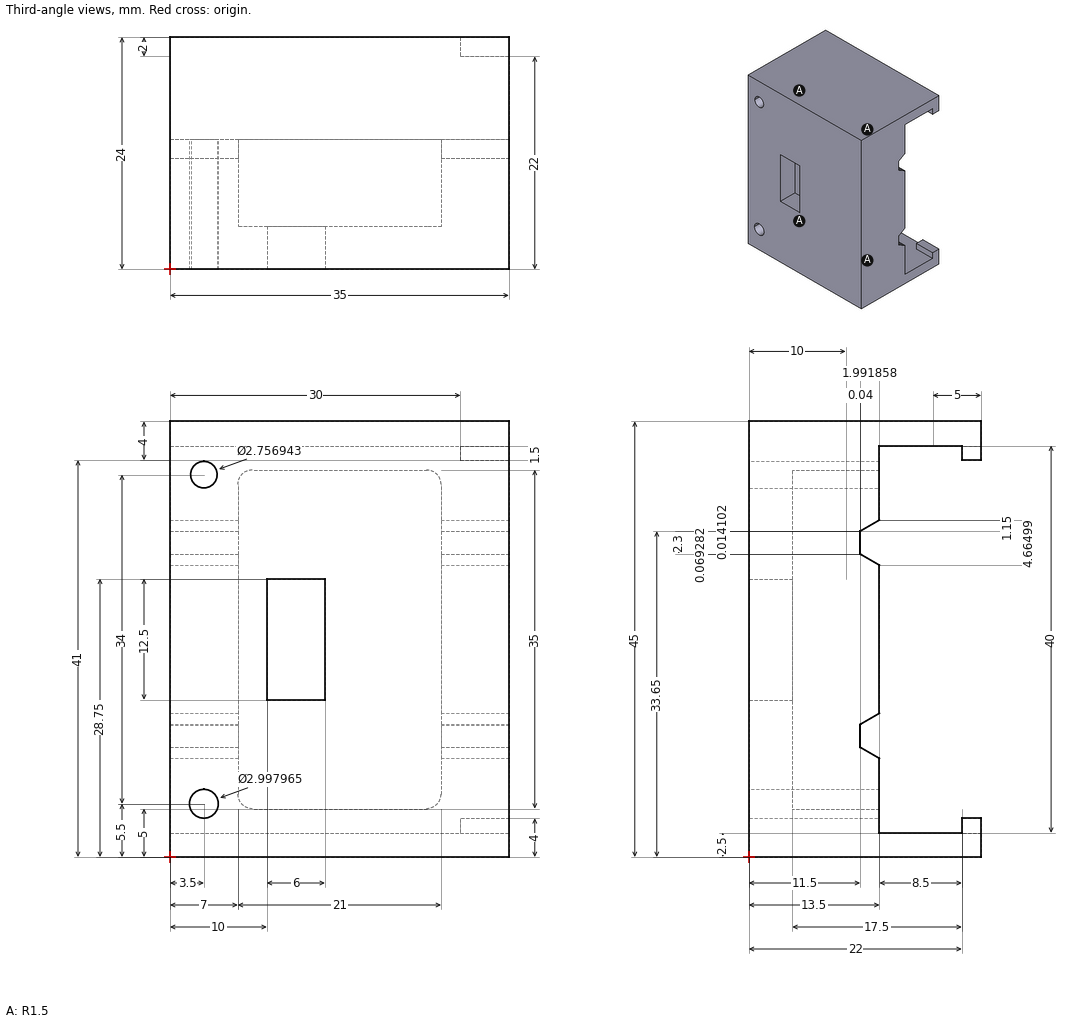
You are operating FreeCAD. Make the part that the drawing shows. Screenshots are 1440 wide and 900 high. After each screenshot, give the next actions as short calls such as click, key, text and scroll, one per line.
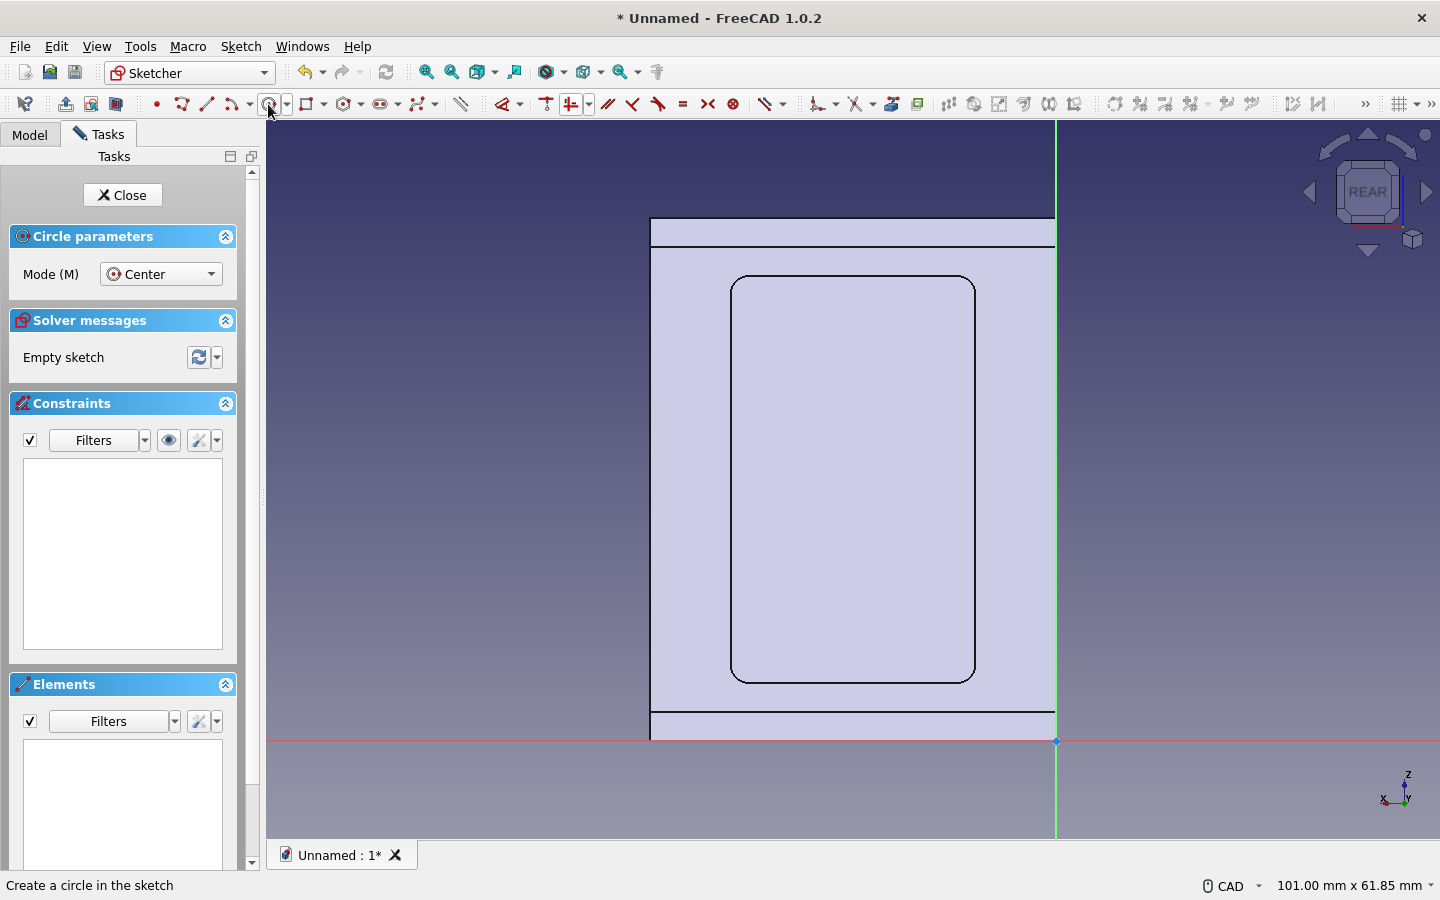
scroll(1016, 677, up, 2)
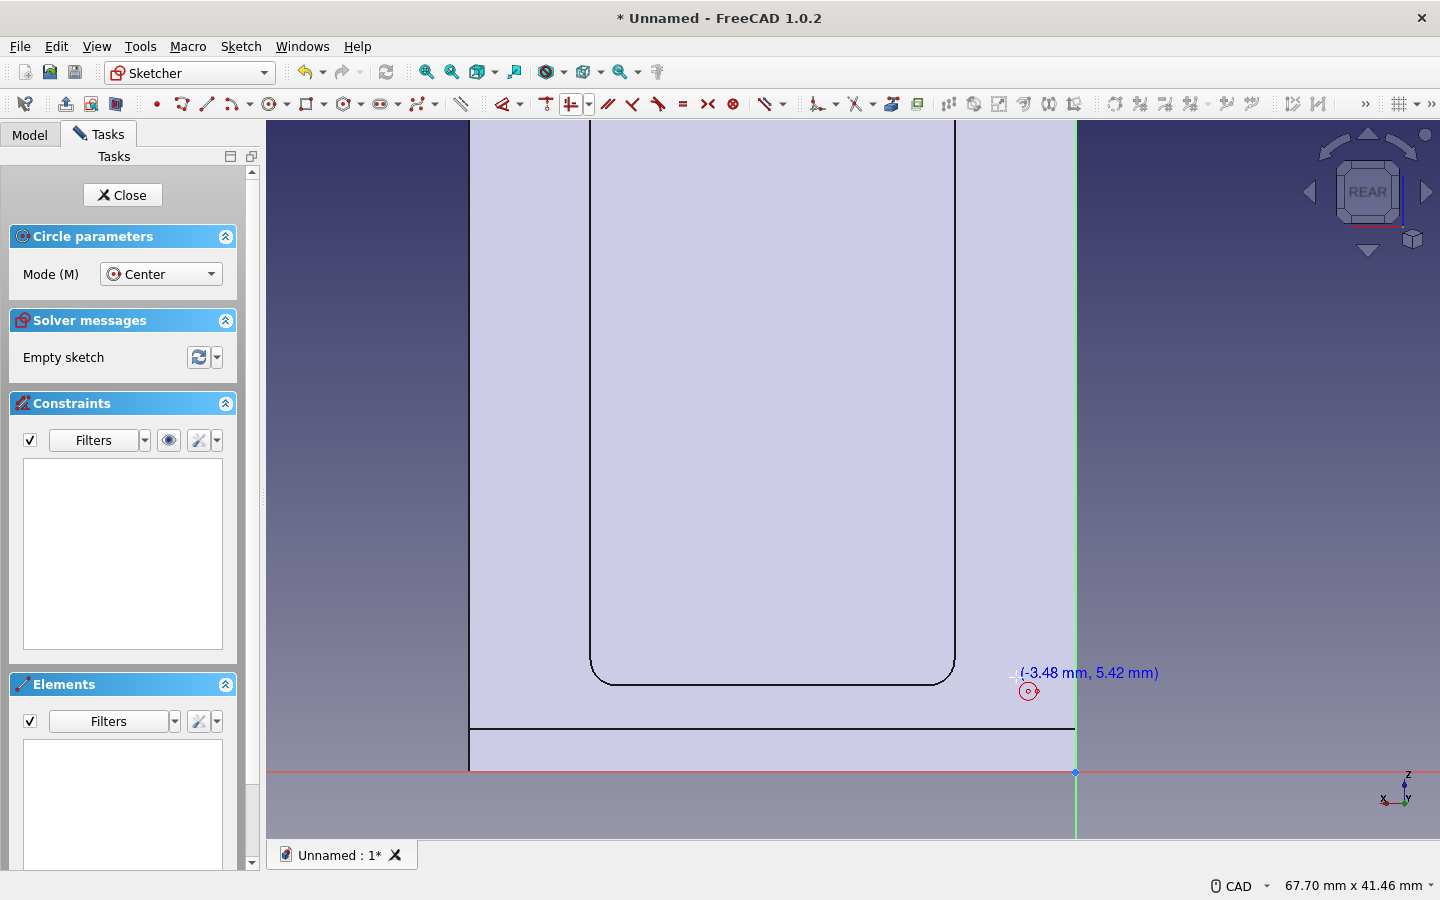
click(1015, 677)
click(1034, 658)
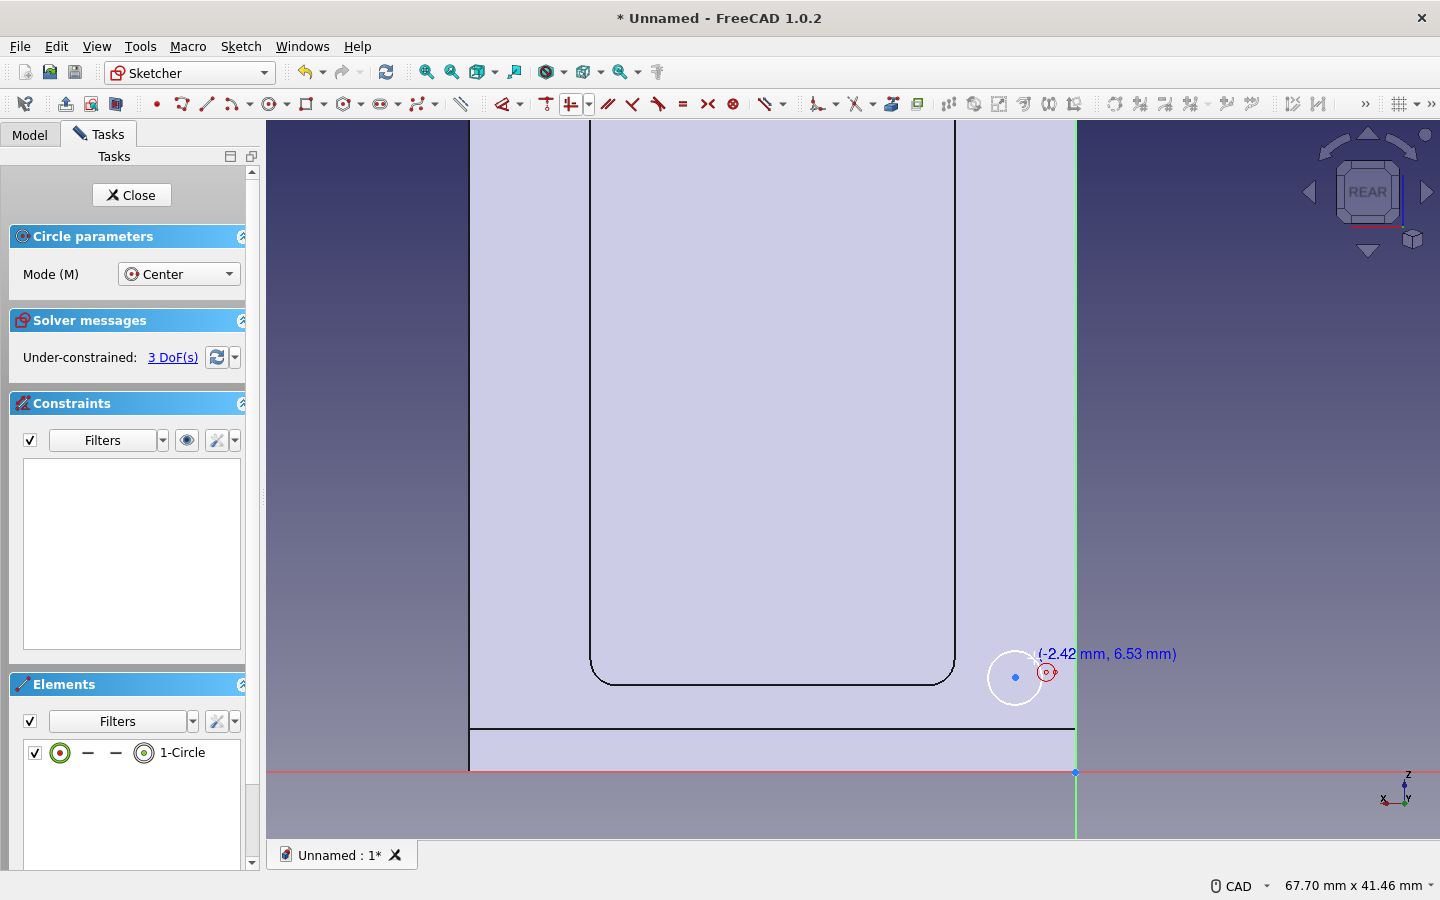
scroll(294, 605, down, 2)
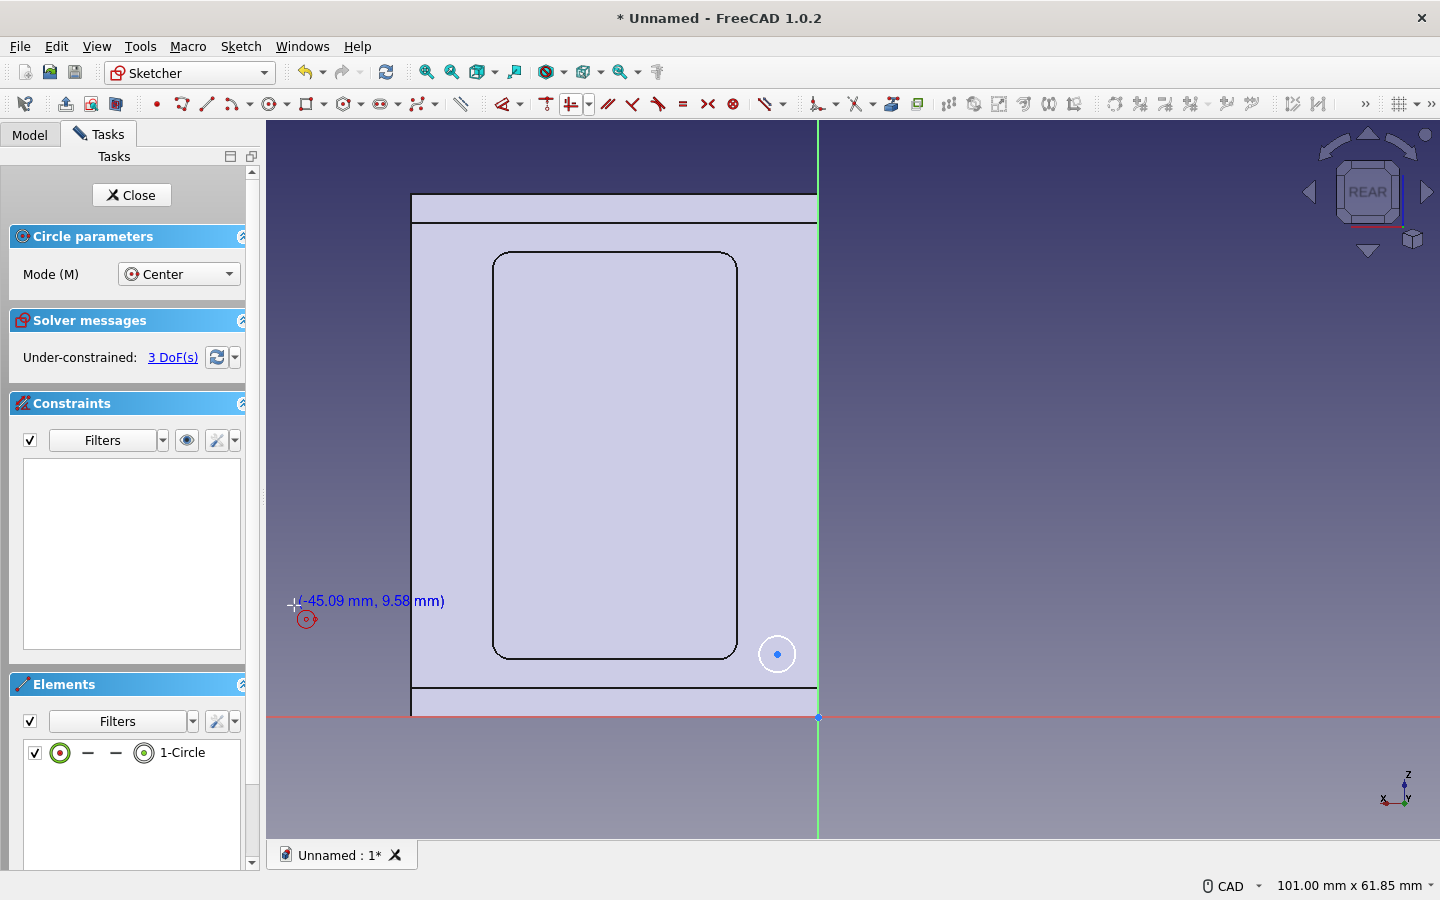
scroll(778, 258, up, 2)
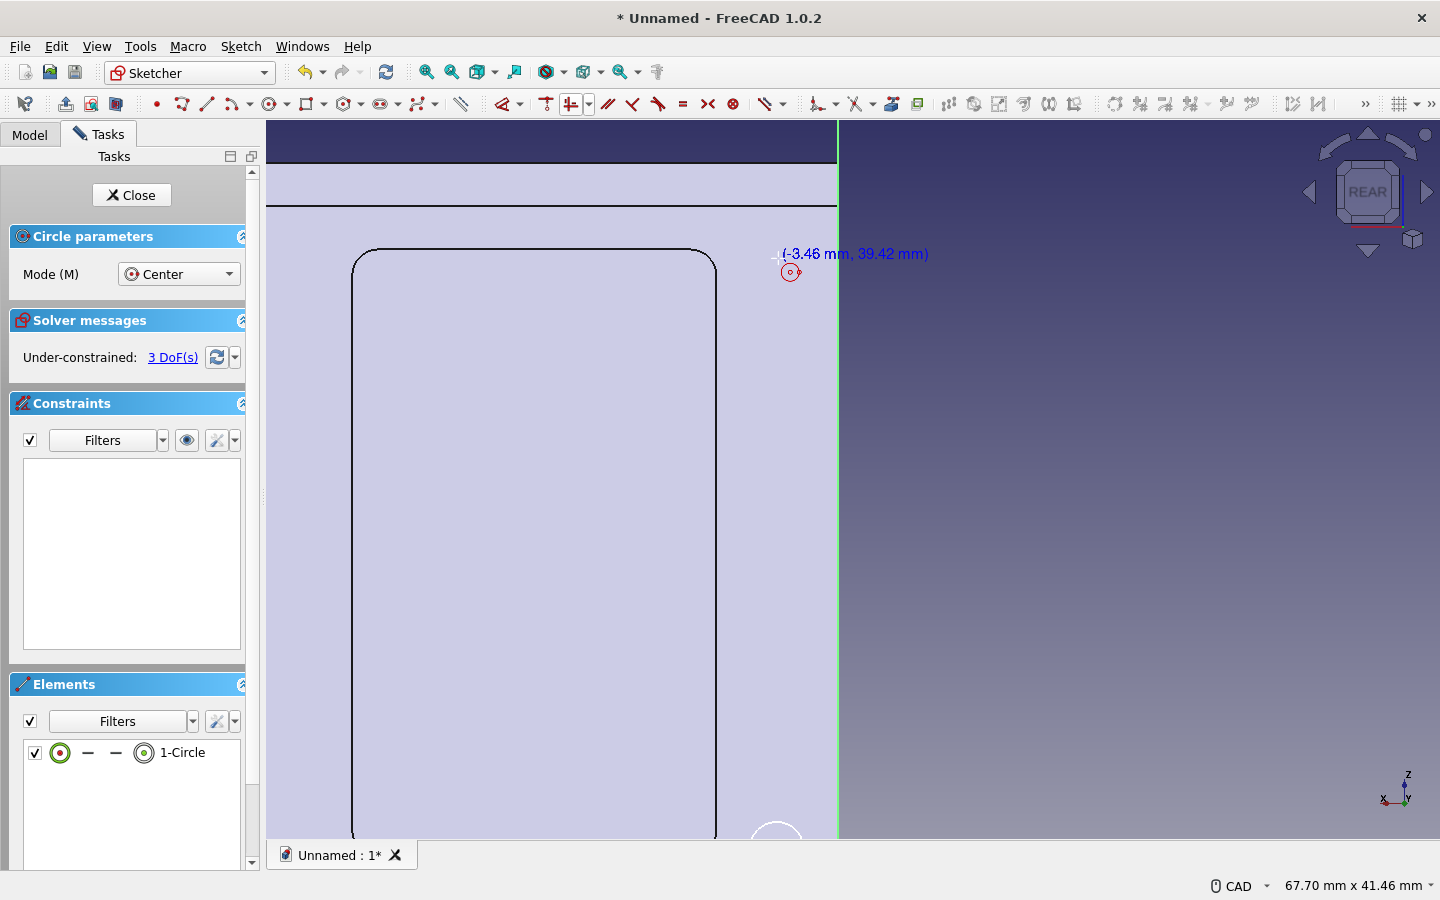
click(777, 258)
click(794, 241)
key(Escape)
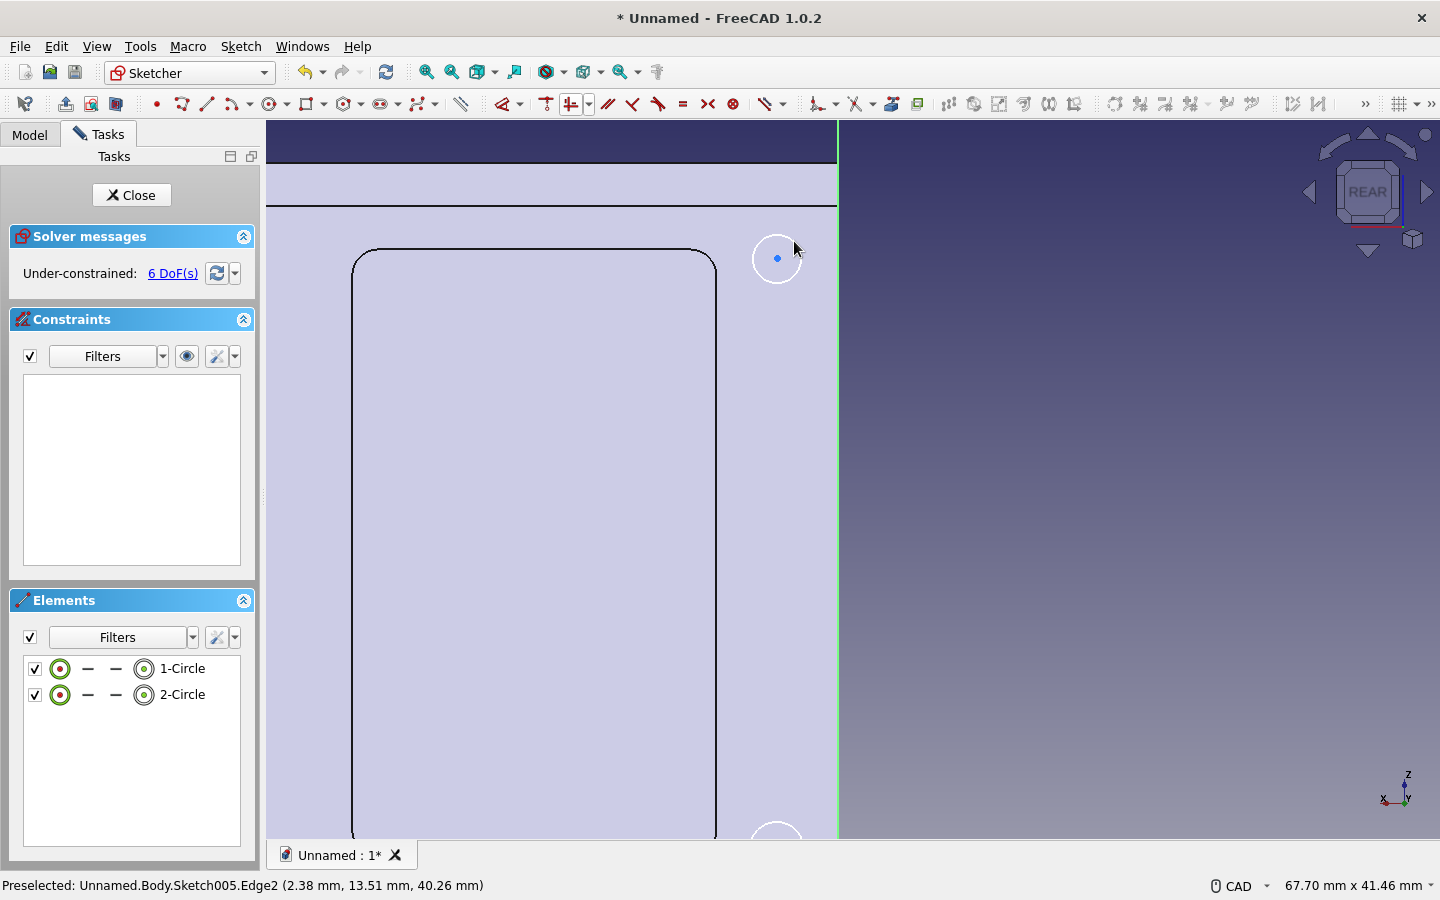
scroll(764, 258, down, 2)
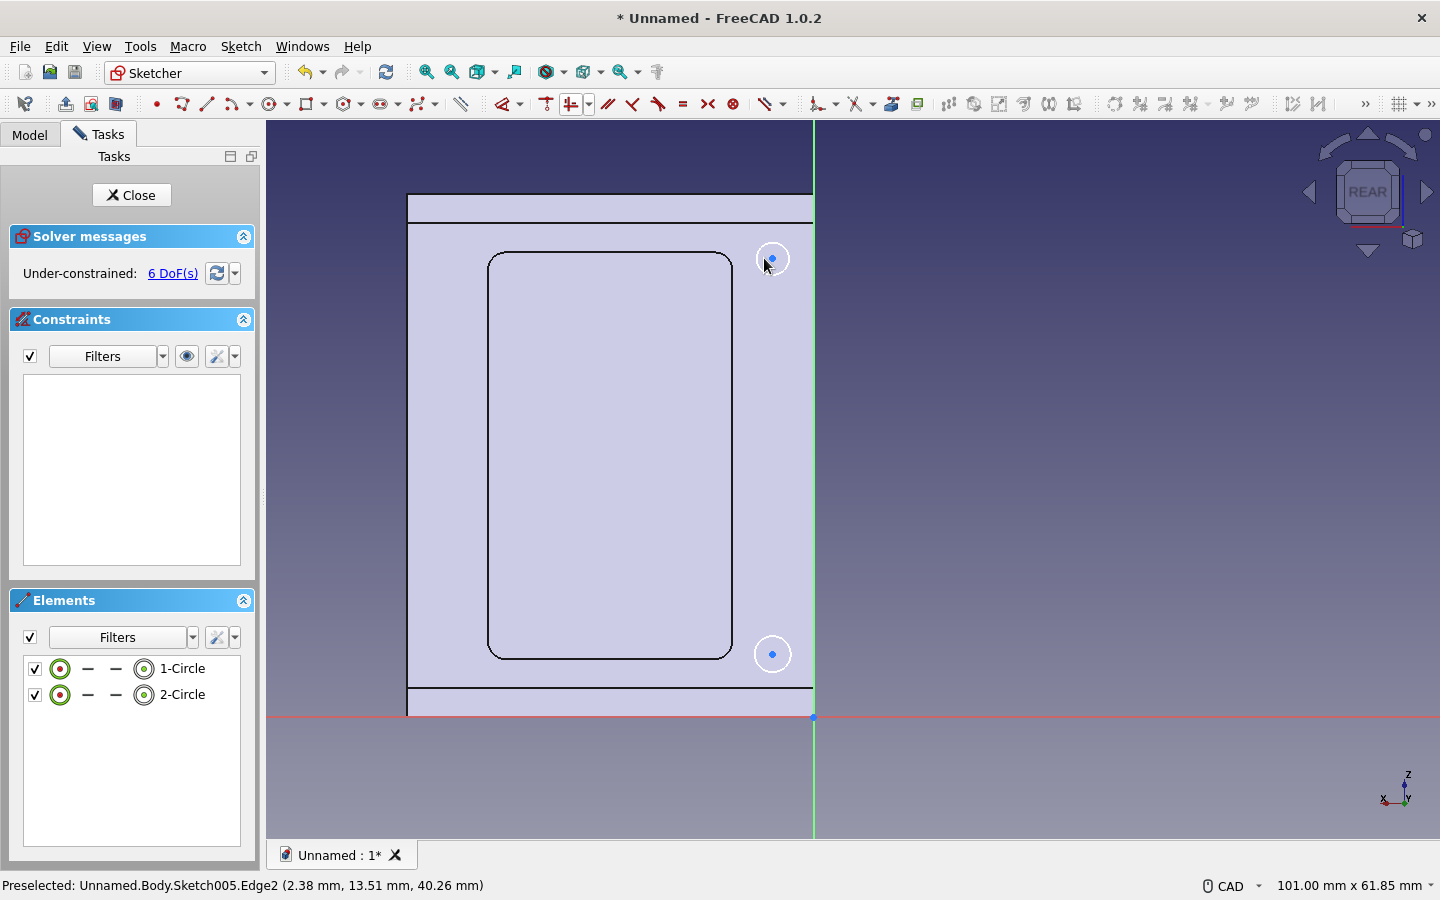
click(773, 654)